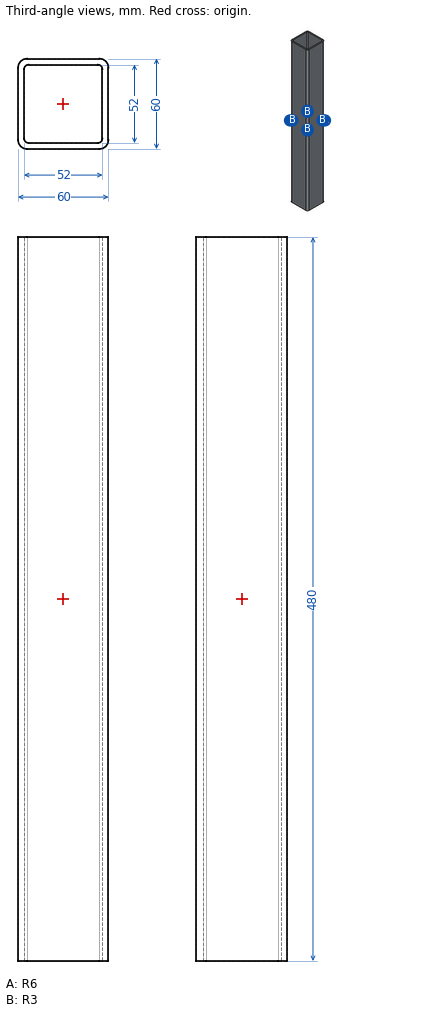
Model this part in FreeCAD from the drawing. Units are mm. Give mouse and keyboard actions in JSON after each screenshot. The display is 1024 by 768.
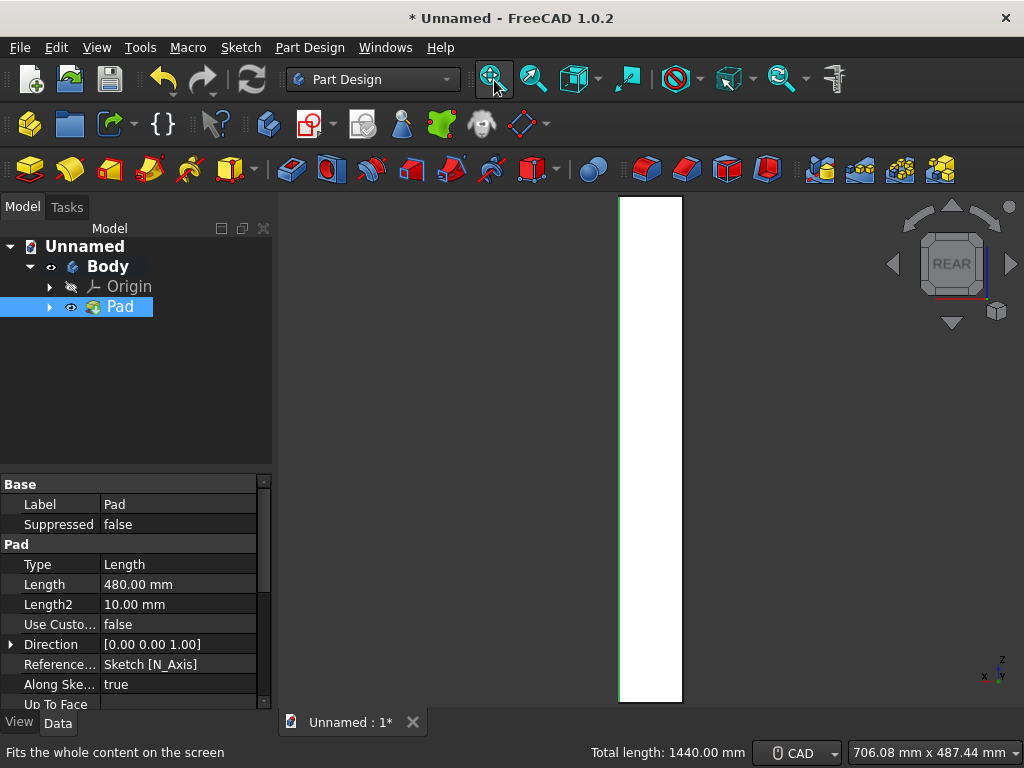
{"action": "left_click", "coordinate": [683, 449], "text": "ctrl"}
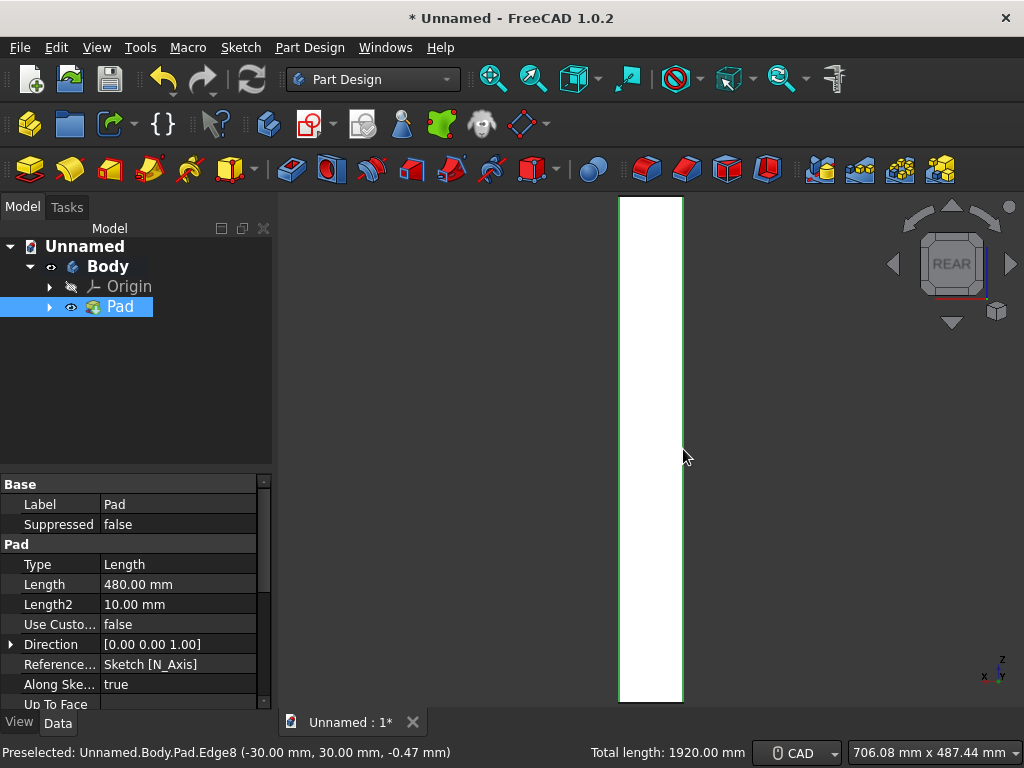
{"action": "left_click", "coordinate": [648, 170]}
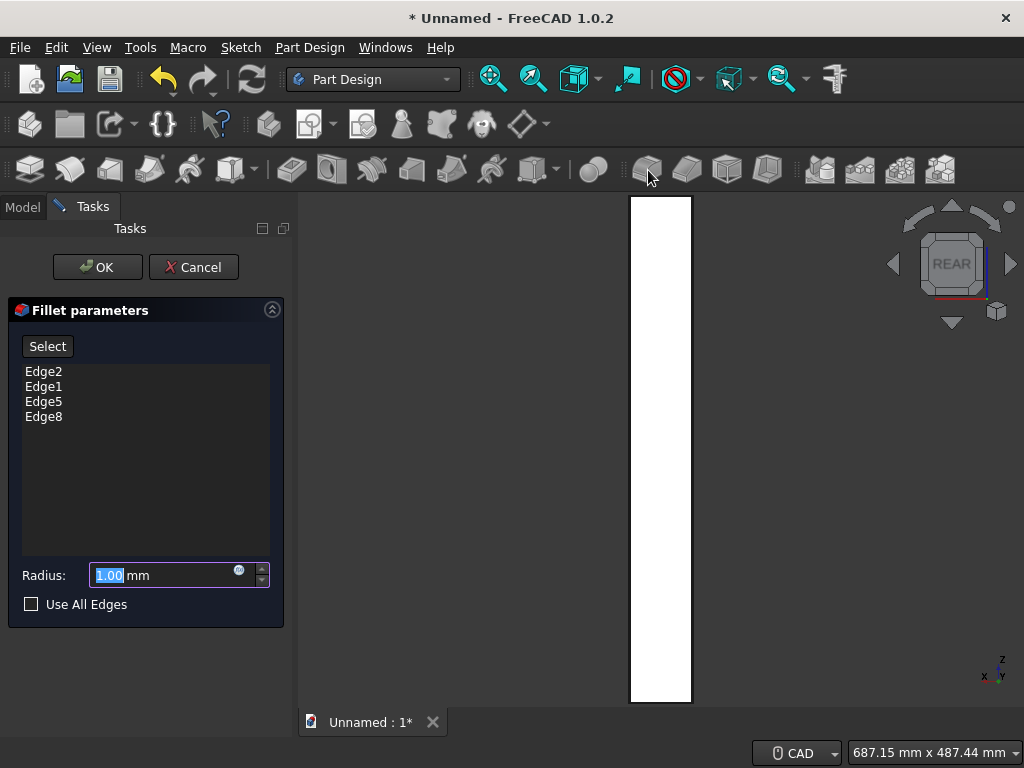
{"action": "type", "text": "6"}
{"action": "key", "text": "Tab"}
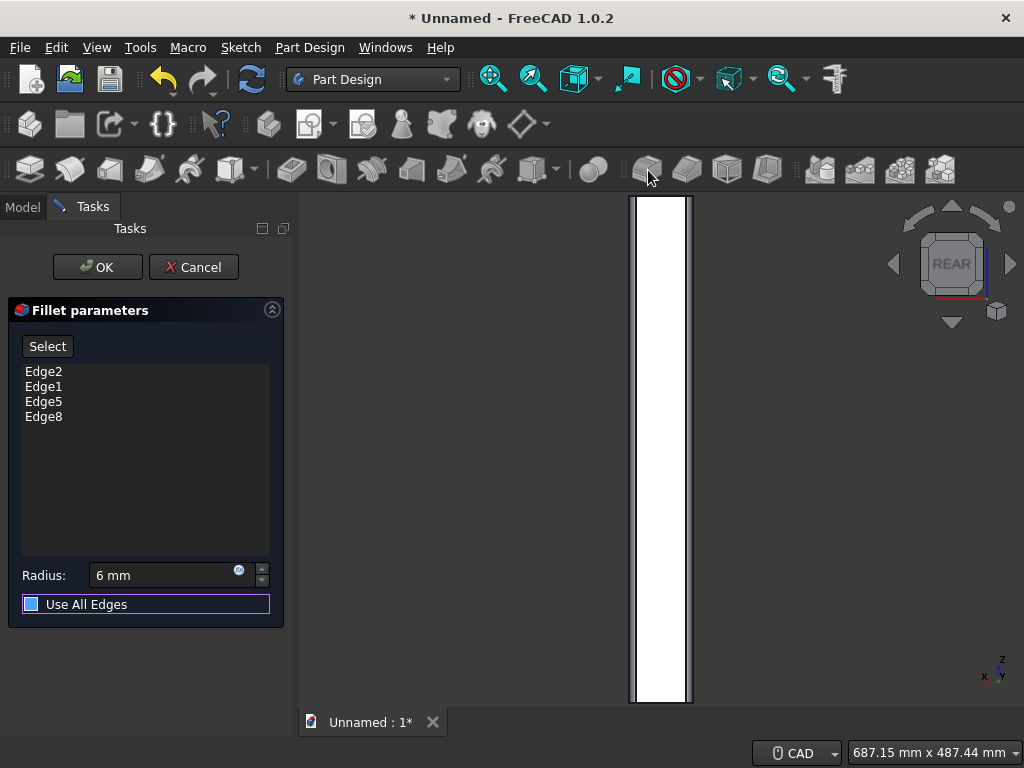
{"action": "left_click", "coordinate": [98, 267]}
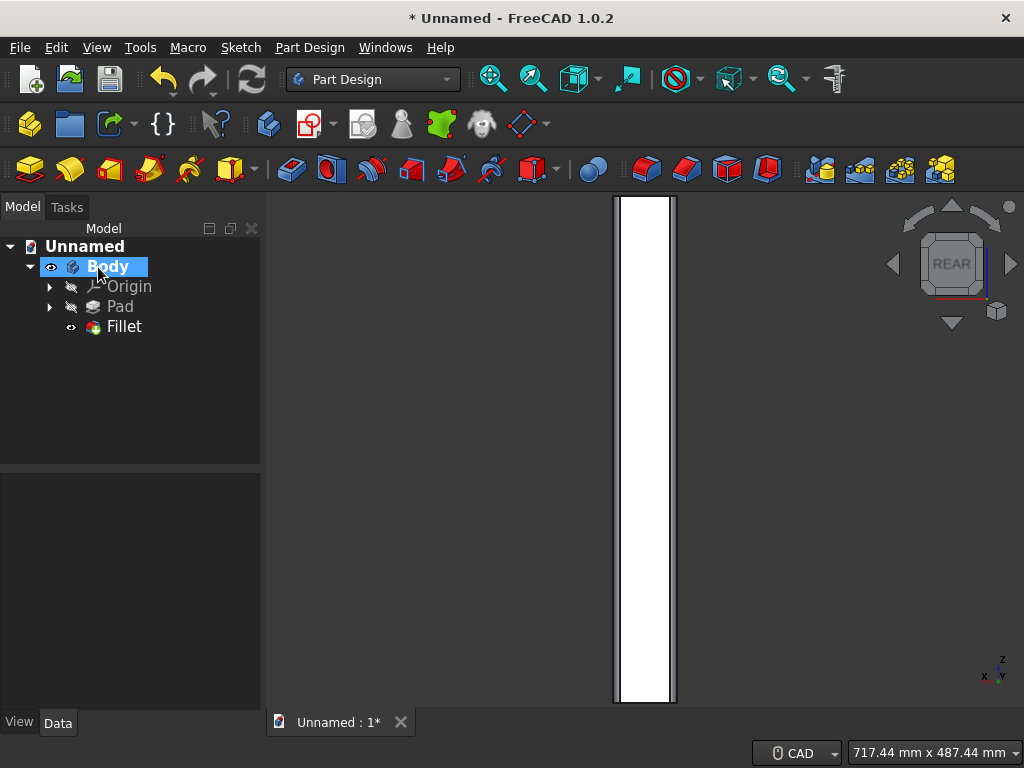
{"action": "key", "text": "0"}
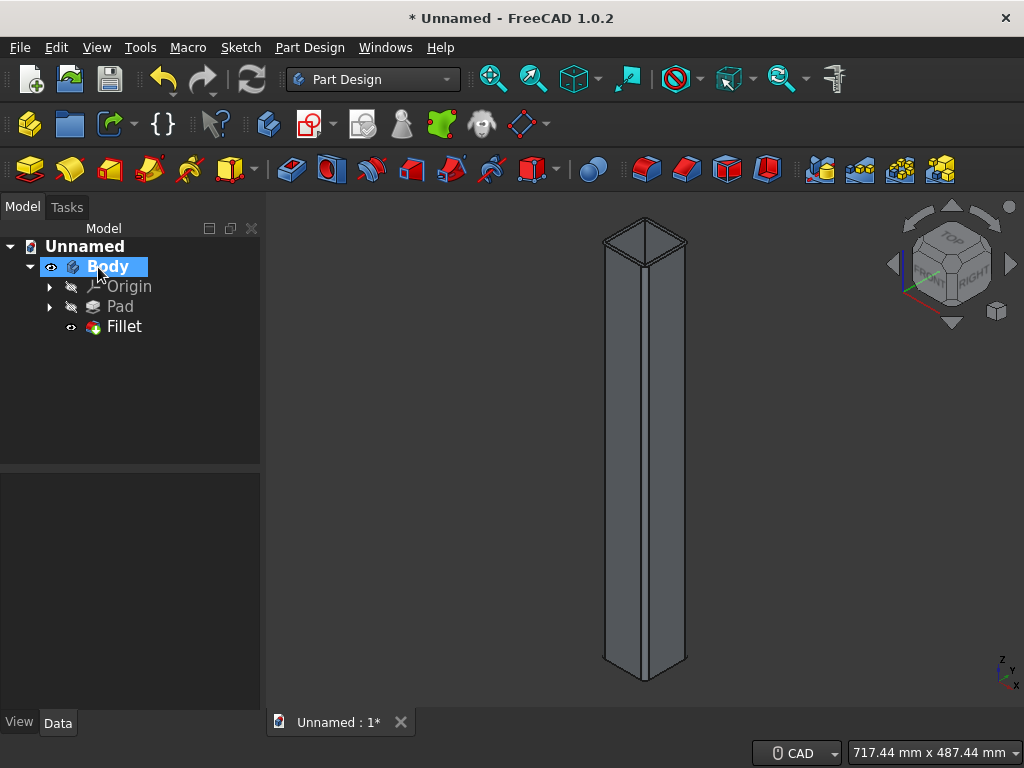
{"action": "key", "text": "2"}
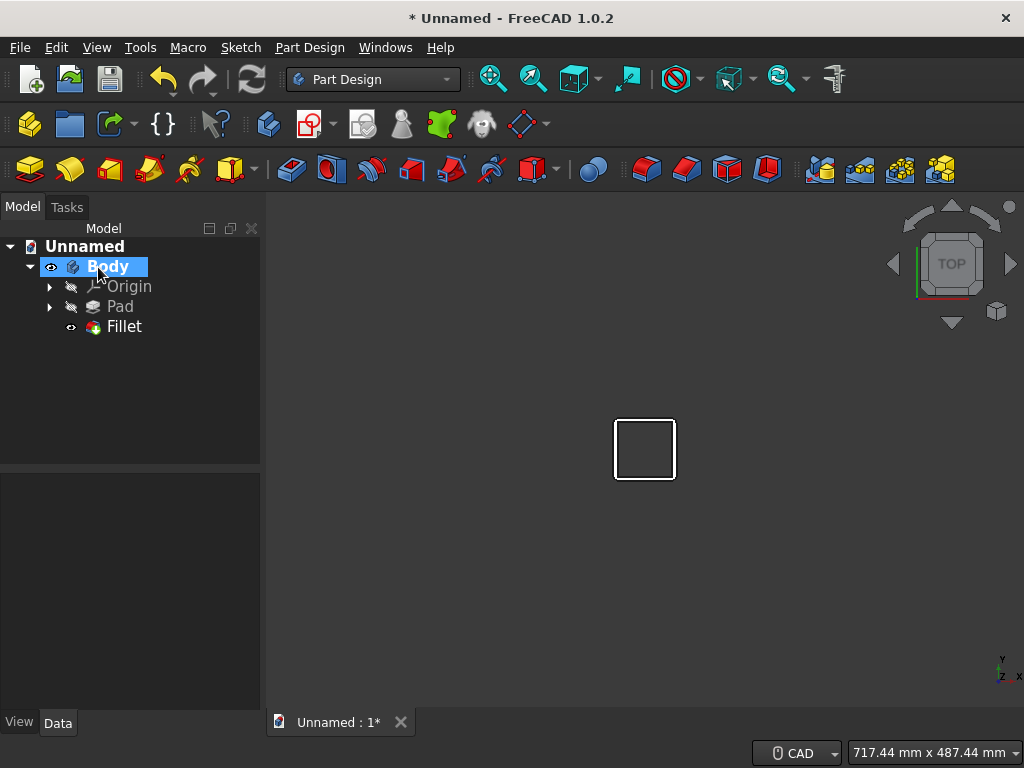
{"action": "left_click", "coordinate": [494, 80]}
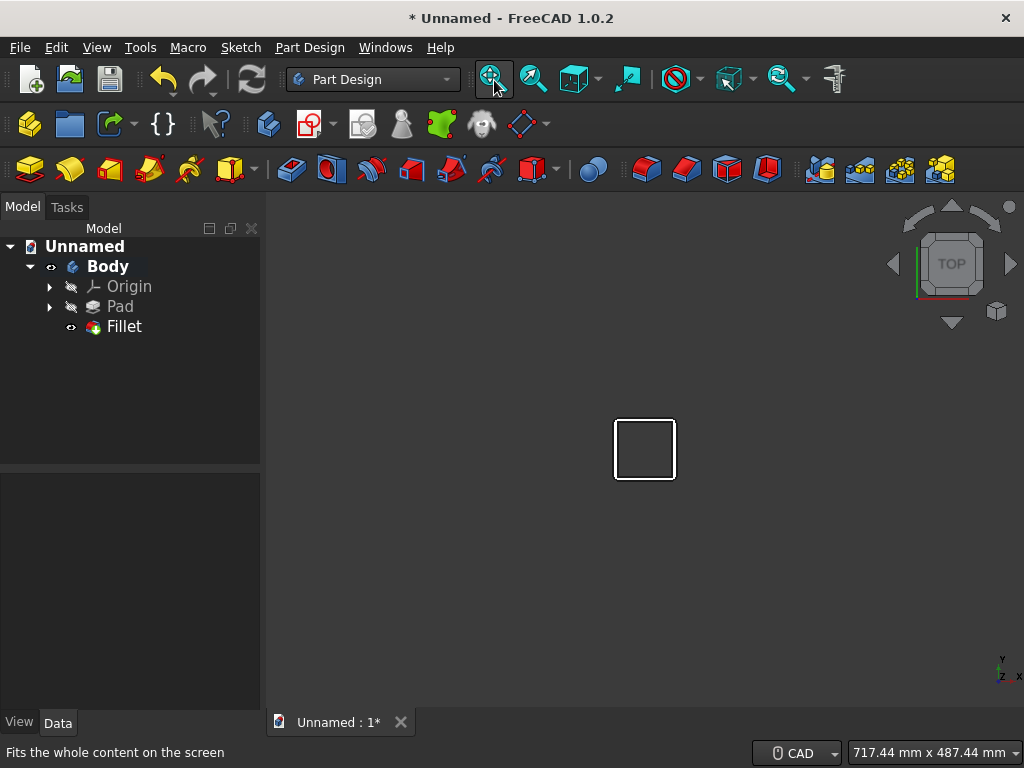
{"action": "key", "text": "1"}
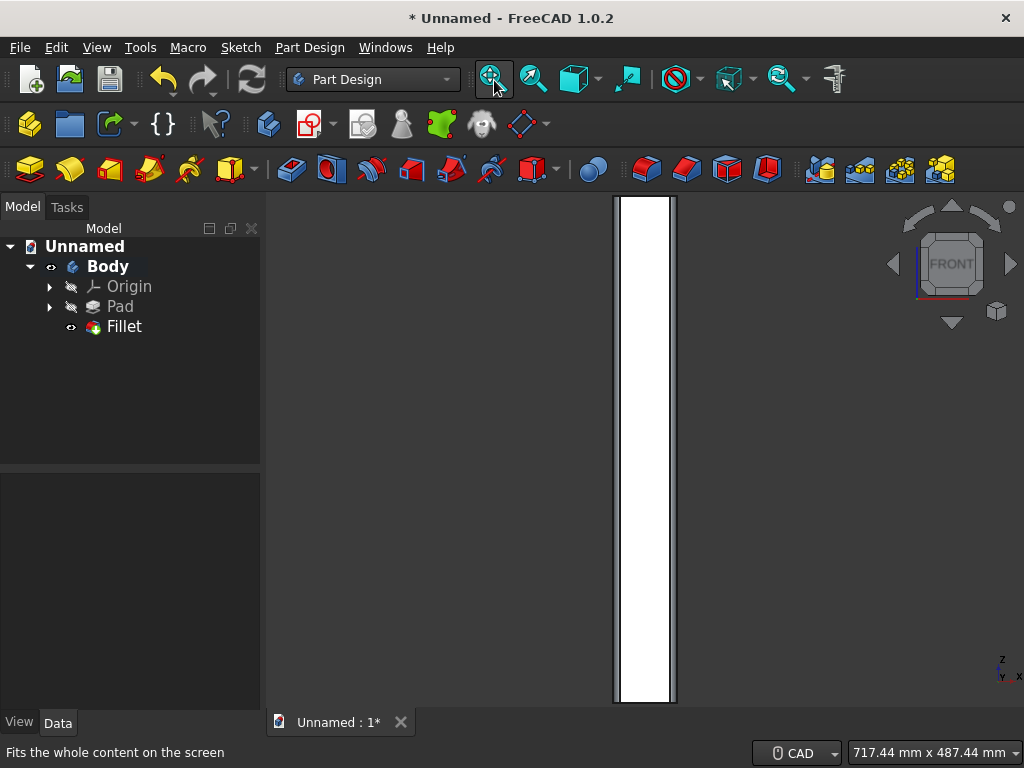
{"action": "key", "text": "3"}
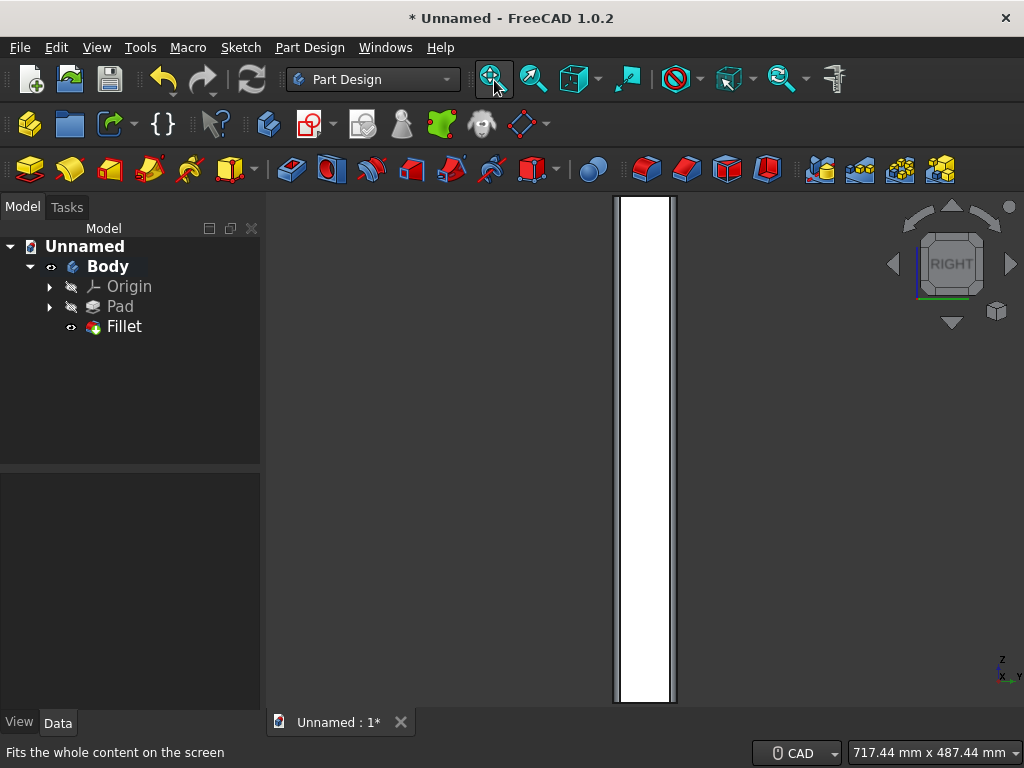
{"action": "key", "text": "5"}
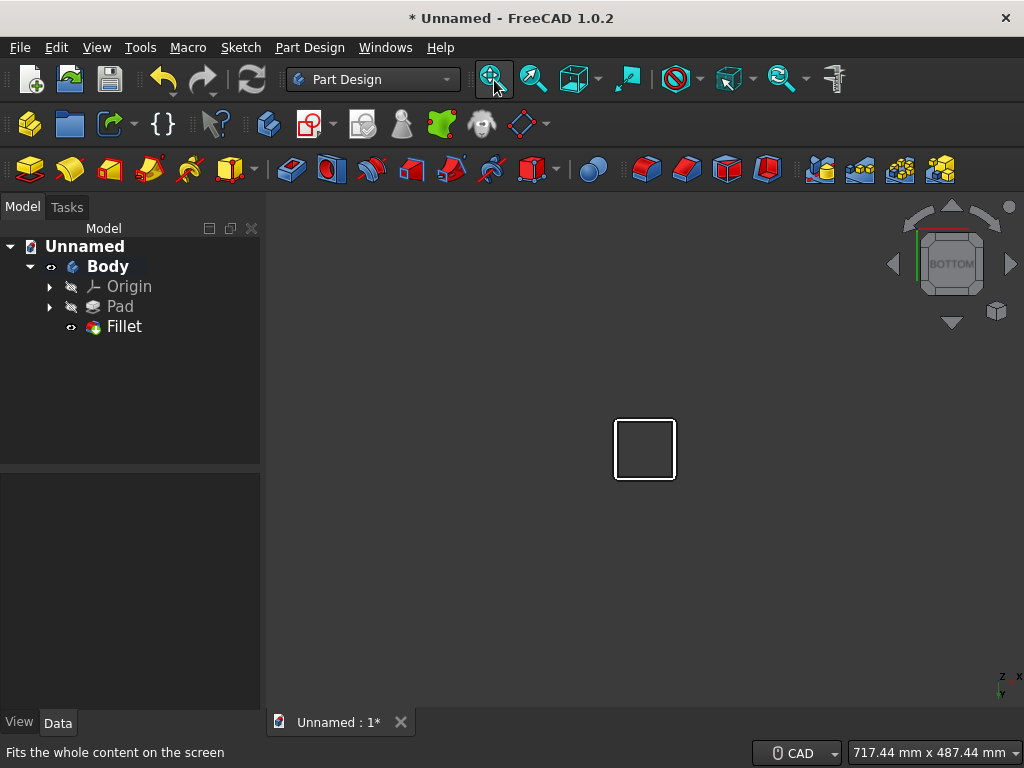
{"action": "left_click", "coordinate": [494, 80]}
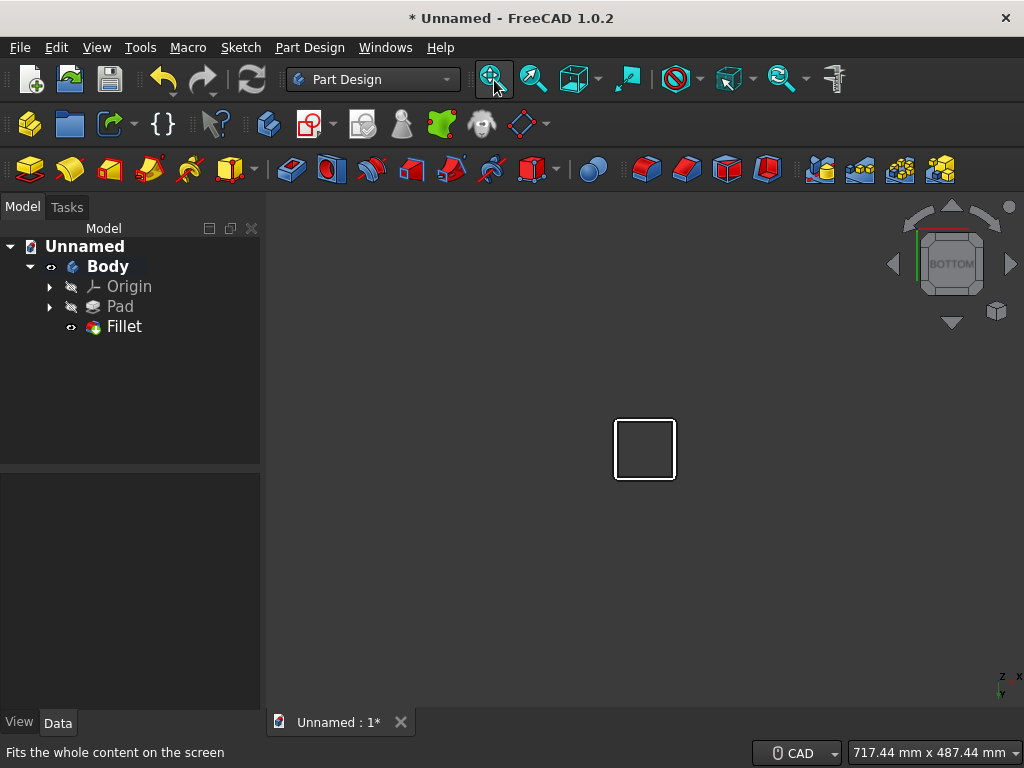
{"action": "key", "text": "4"}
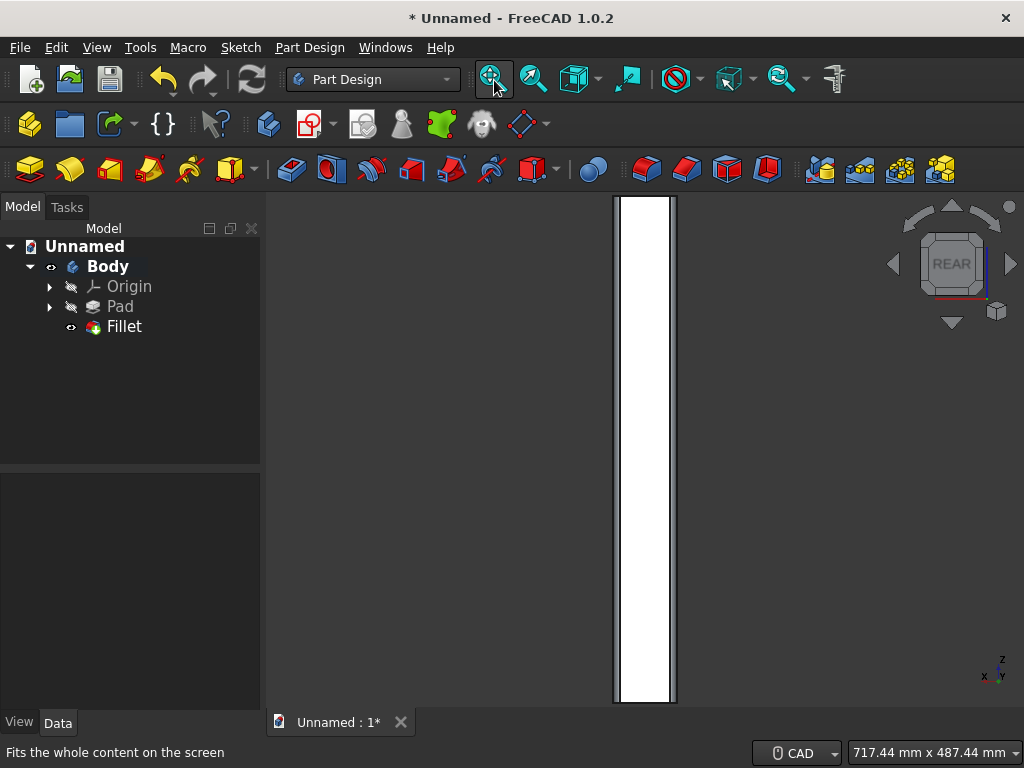
{"action": "key", "text": "6"}